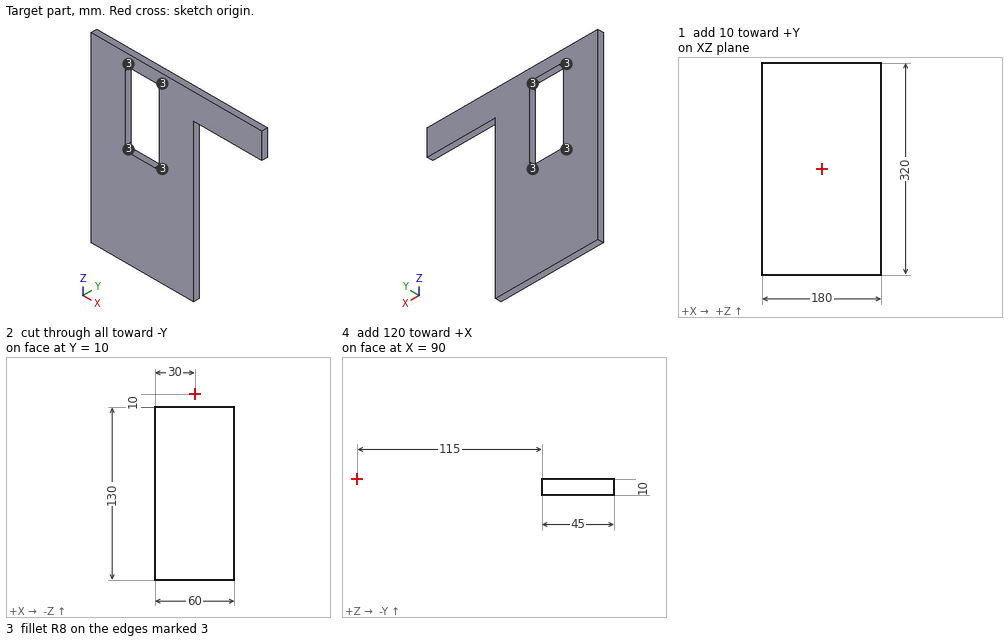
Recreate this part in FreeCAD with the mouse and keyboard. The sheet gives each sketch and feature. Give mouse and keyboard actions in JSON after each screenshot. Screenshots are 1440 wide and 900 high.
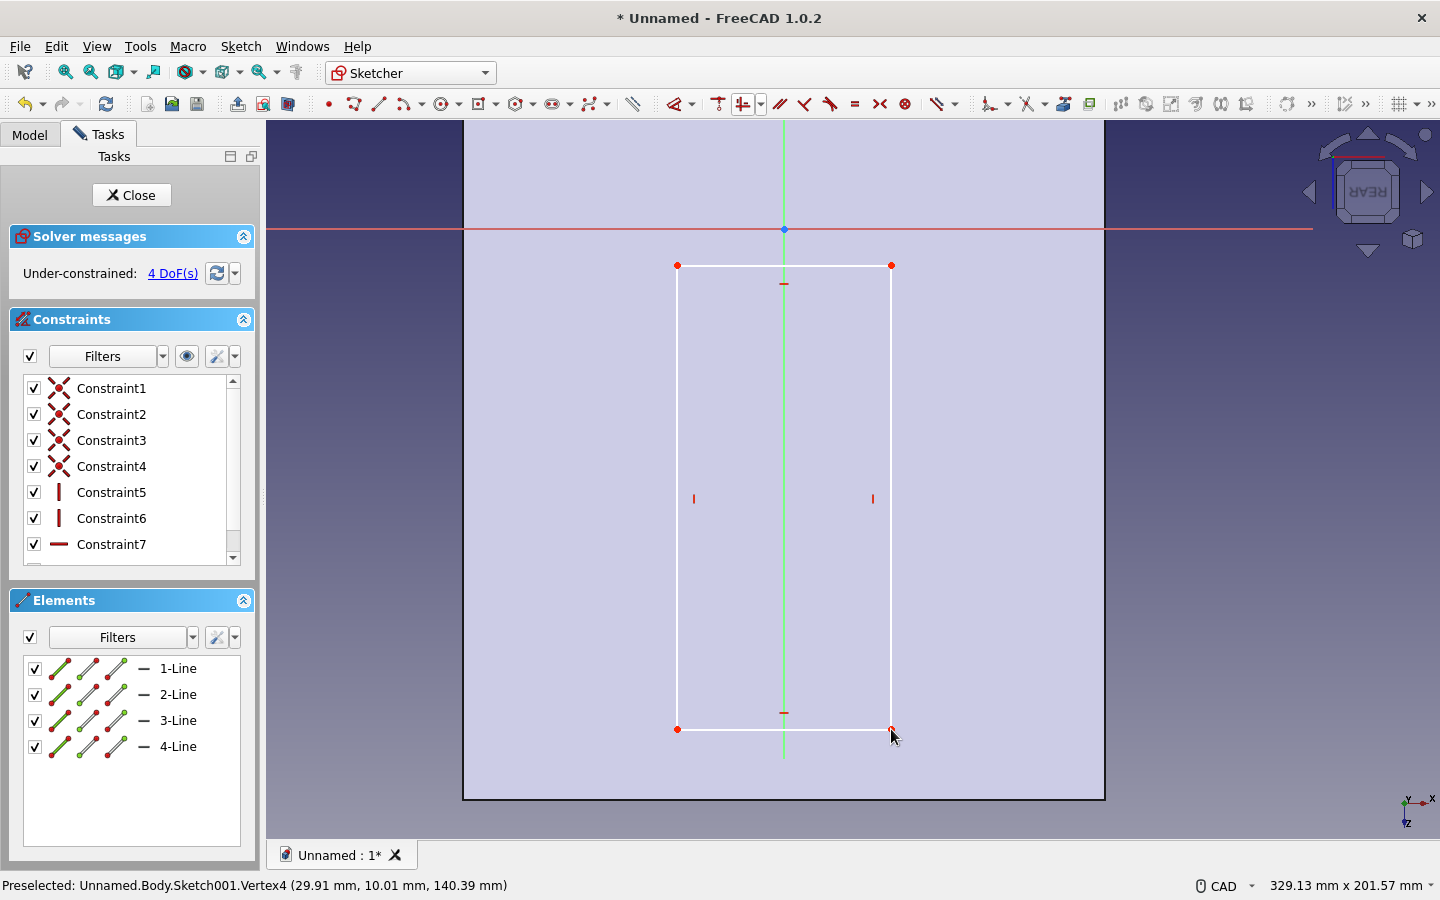
{"action": "key", "text": "d"}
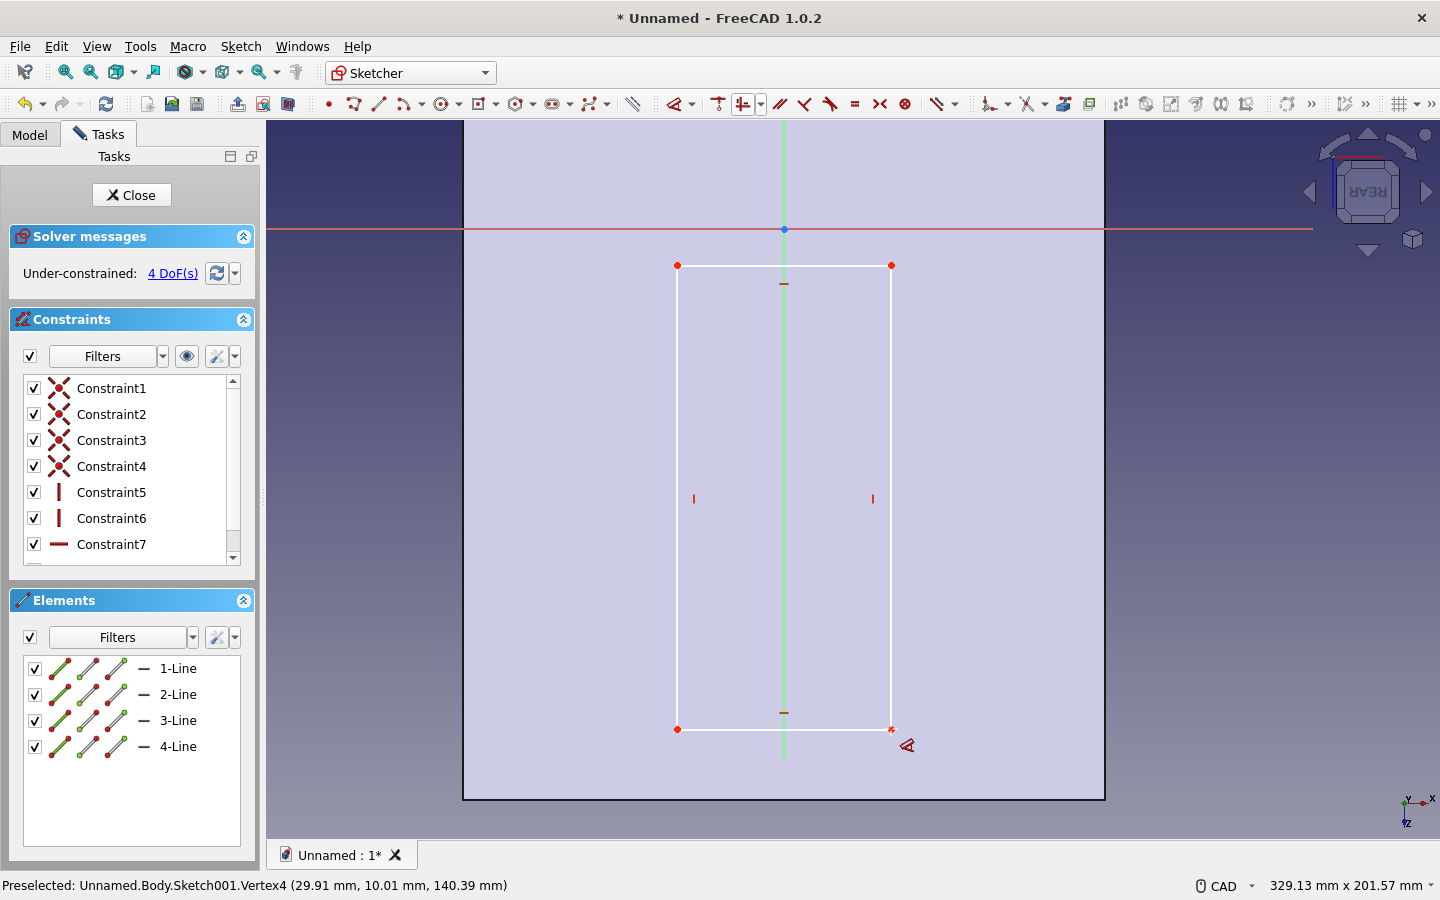
{"action": "left_click", "coordinate": [741, 730]}
{"action": "left_click", "coordinate": [735, 764]}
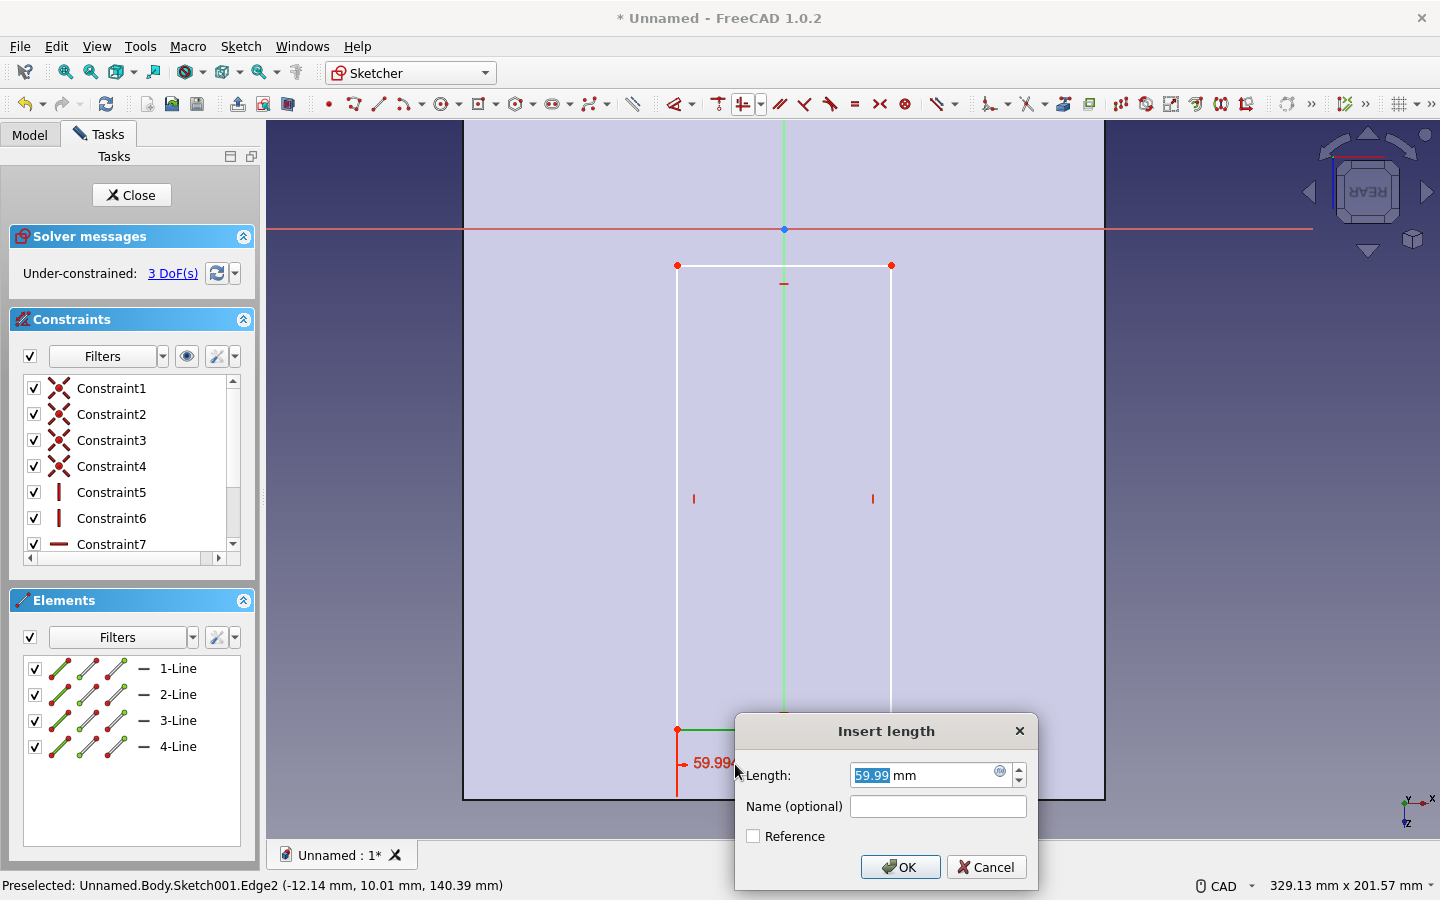
{"action": "type", "text": "60"}
{"action": "key", "text": "Return"}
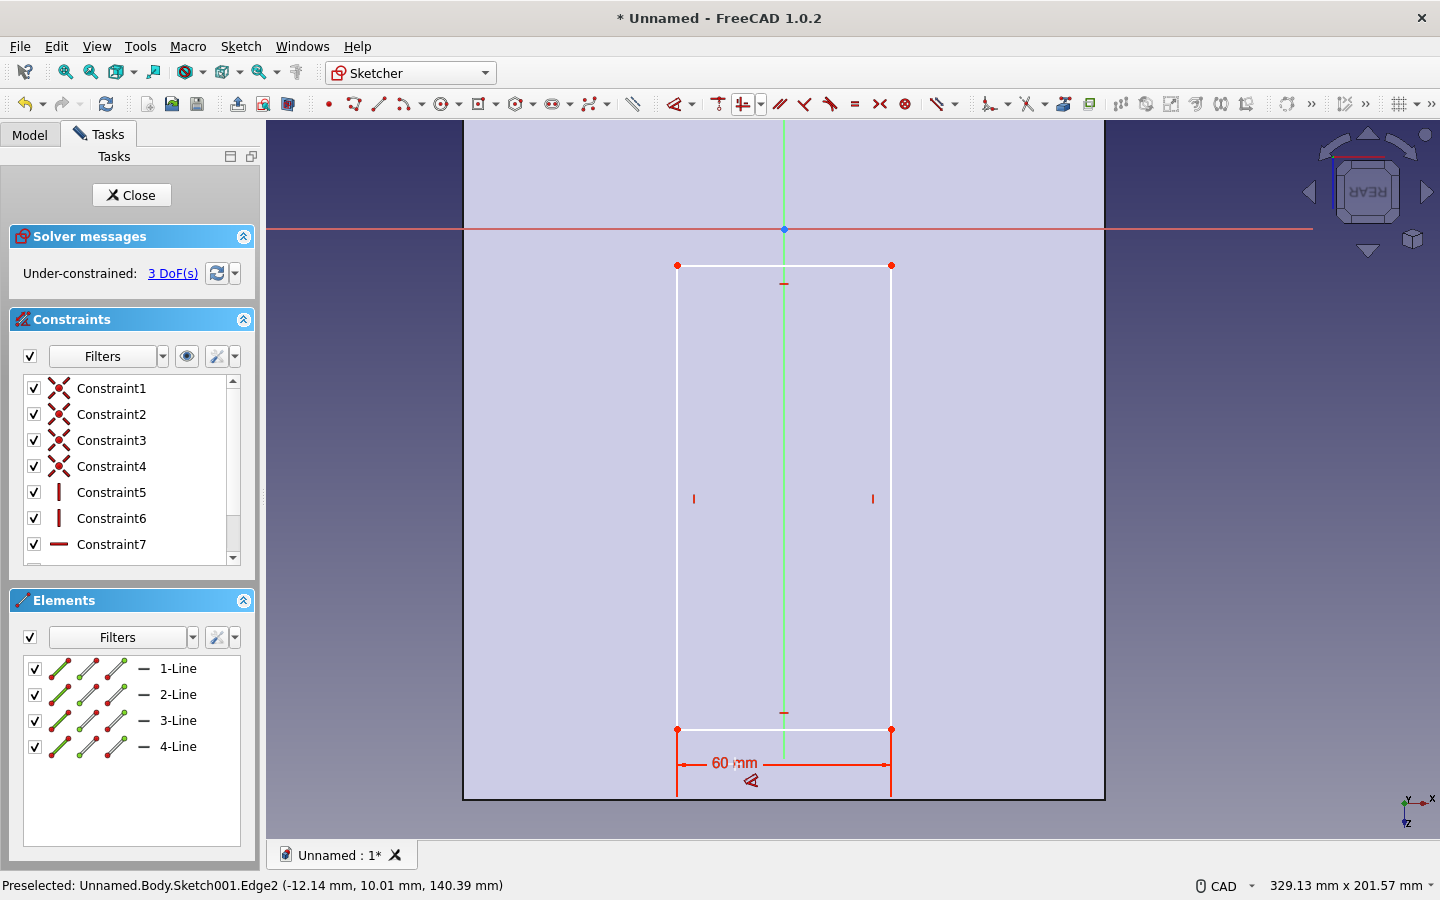
{"action": "left_click", "coordinate": [677, 405]}
{"action": "left_click", "coordinate": [643, 498]}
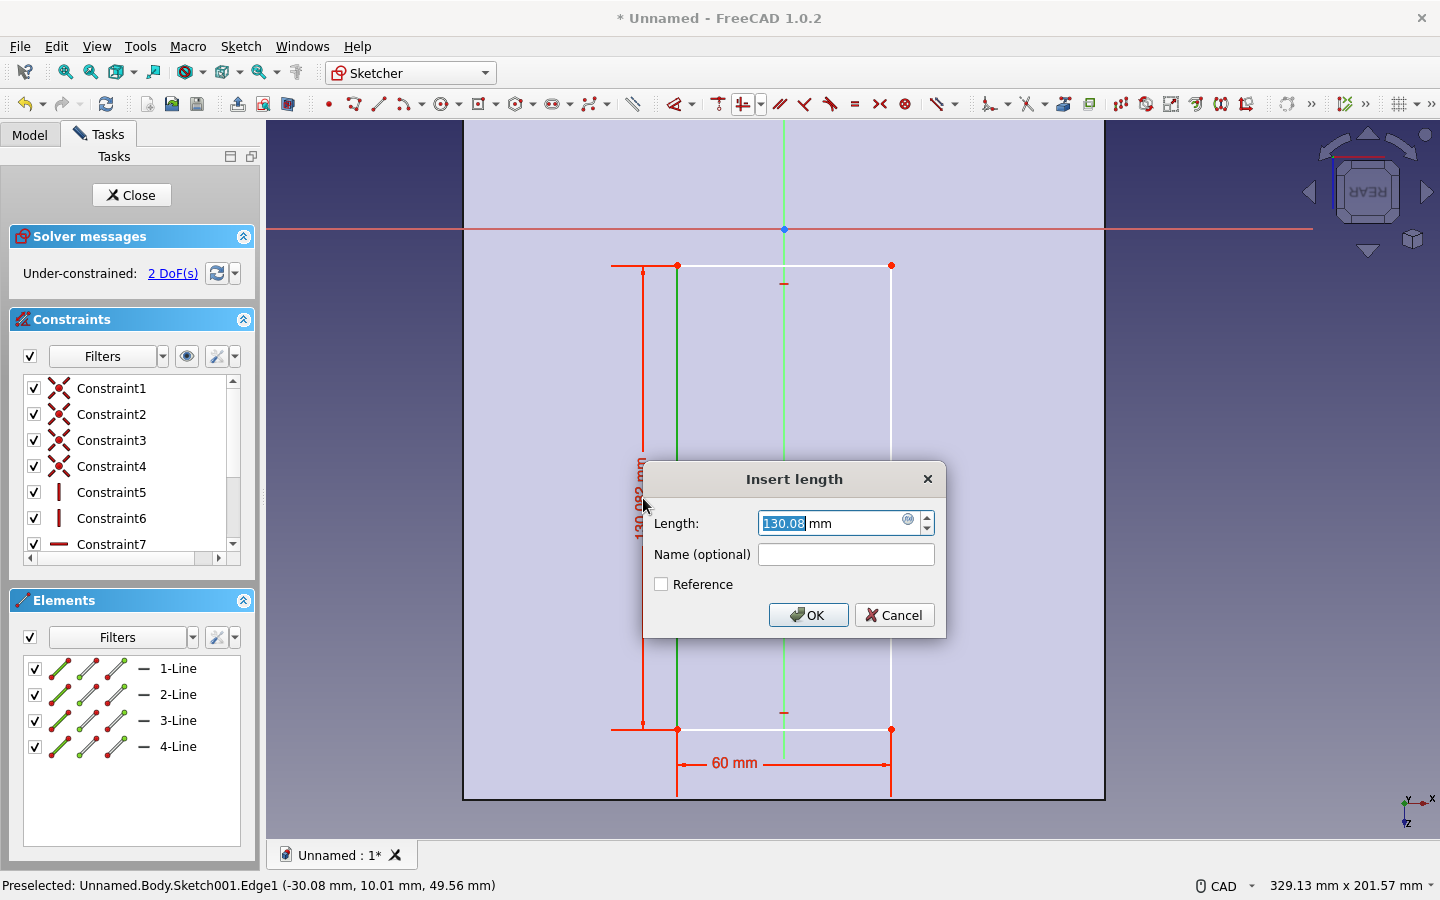
{"action": "type", "text": "130"}
{"action": "key", "text": "Return"}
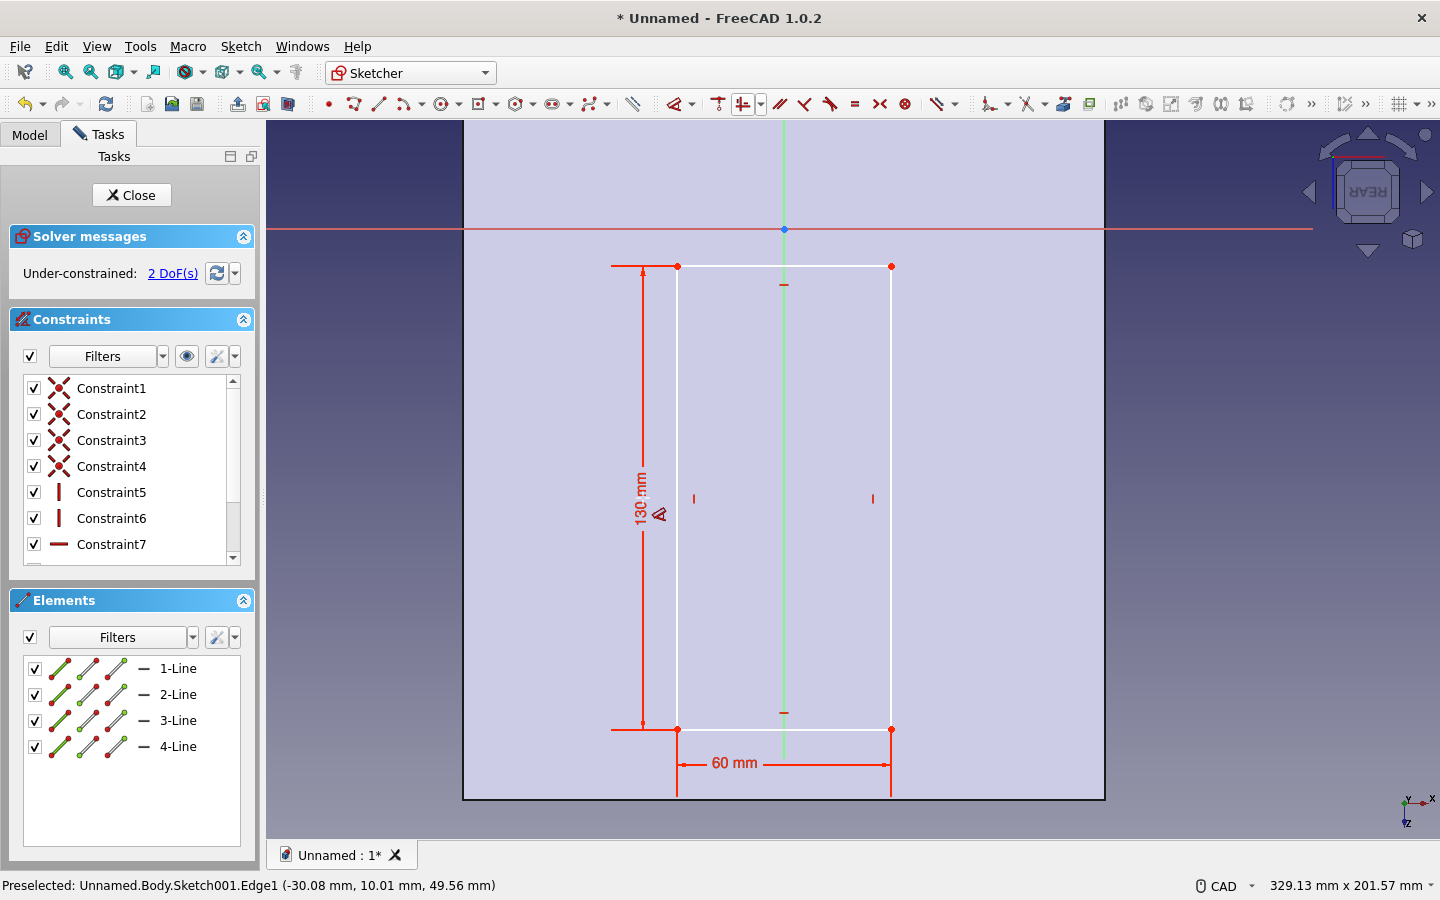
{"action": "left_click", "coordinate": [677, 266]}
{"action": "left_click", "coordinate": [731, 195]}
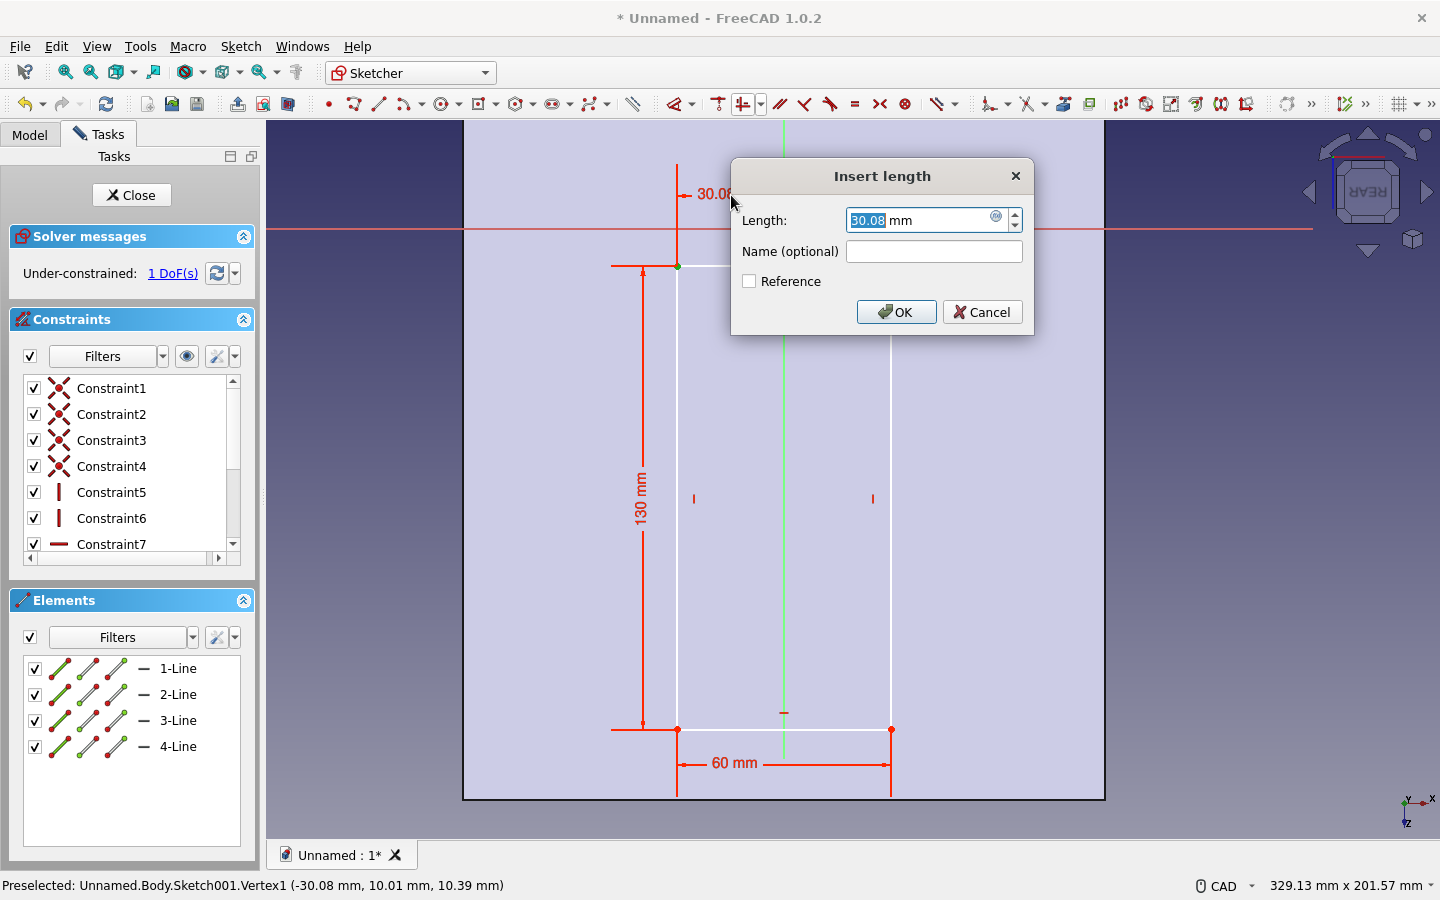
{"action": "type", "text": "30"}
{"action": "key", "text": "Return"}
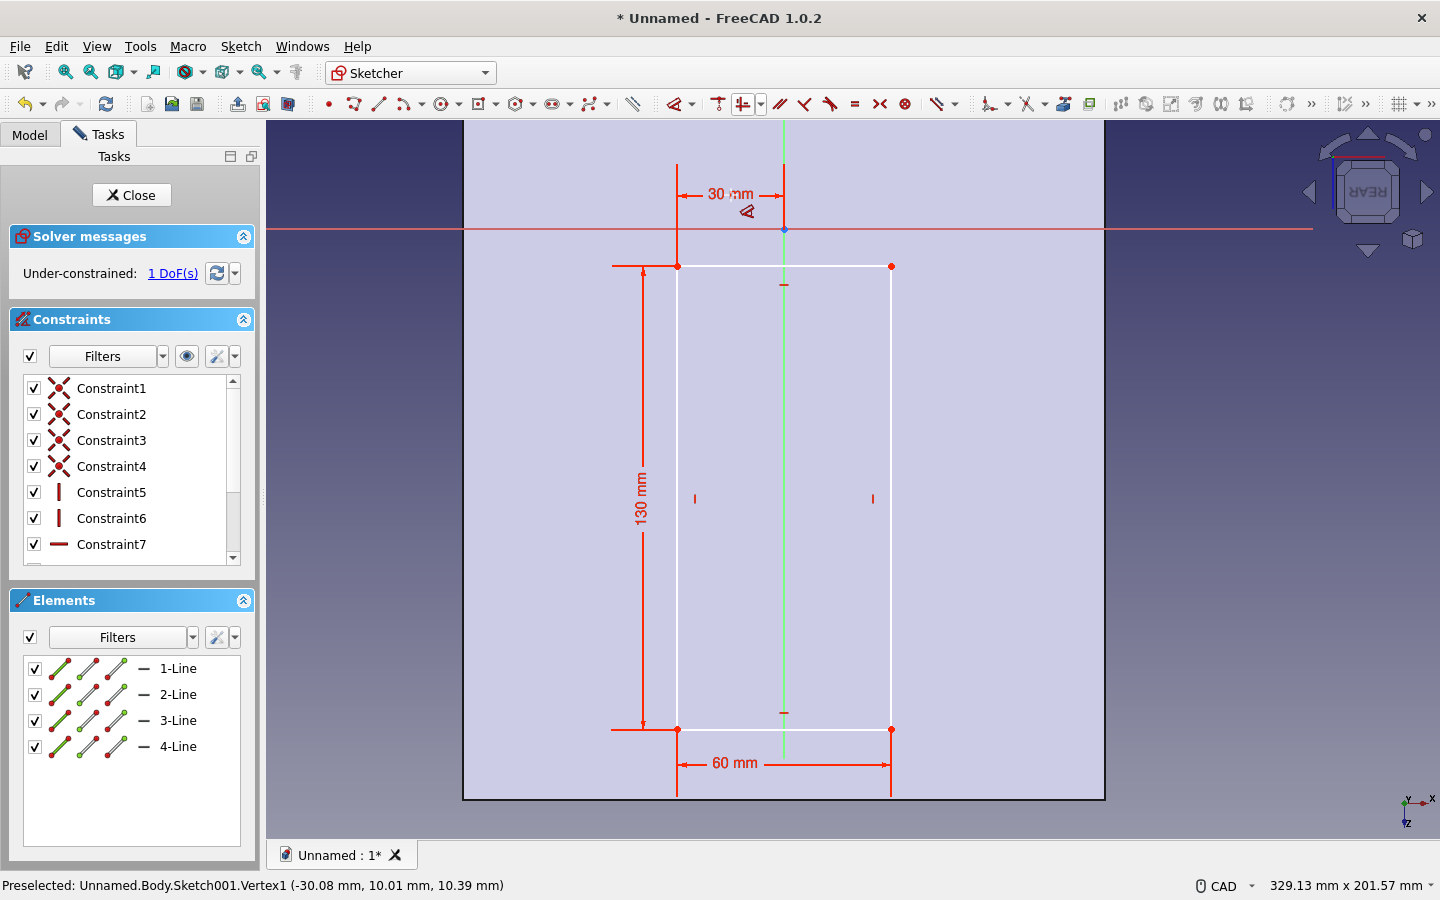
{"action": "left_click", "coordinate": [677, 266]}
{"action": "left_click", "coordinate": [643, 248]}